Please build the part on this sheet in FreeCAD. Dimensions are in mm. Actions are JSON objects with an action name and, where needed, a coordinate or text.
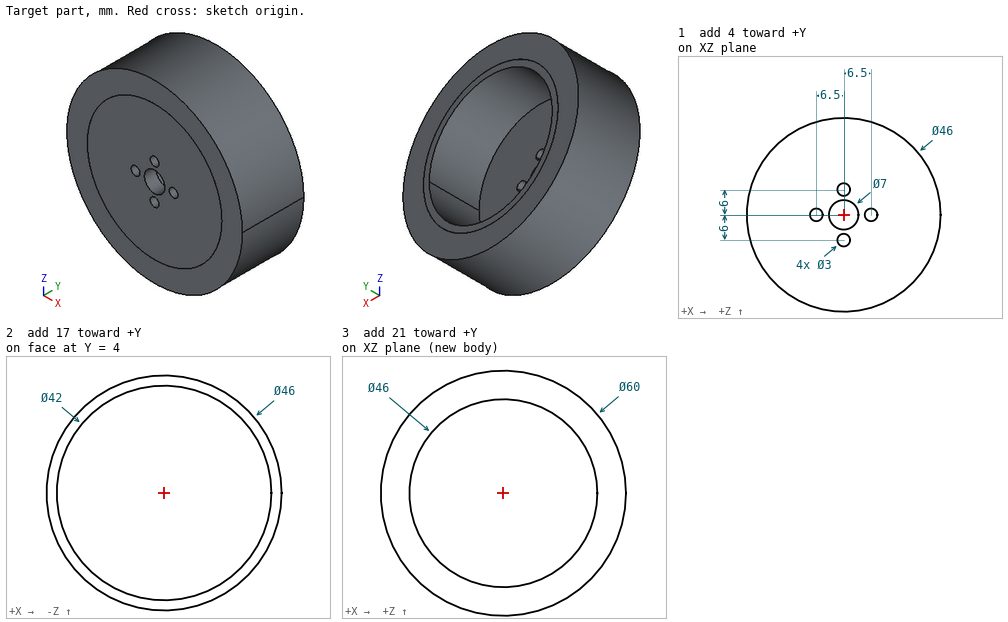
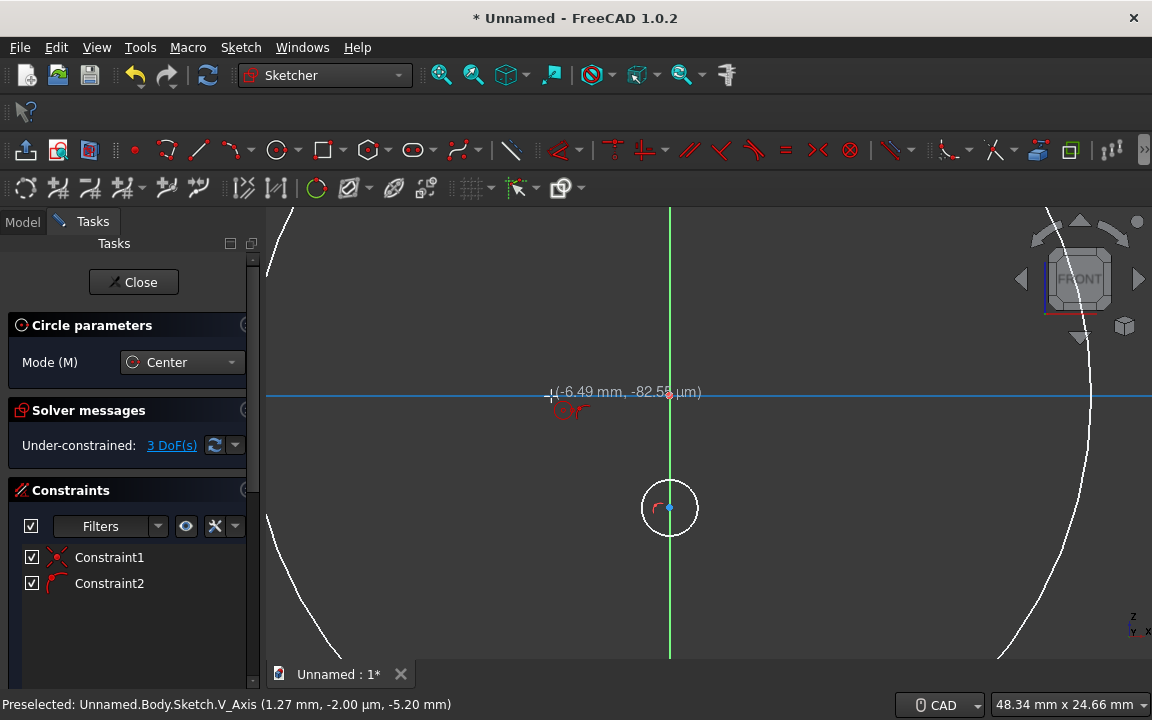
{"action": "scroll", "coordinate": [628, 449], "scroll_direction": "down", "scroll_amount": 6}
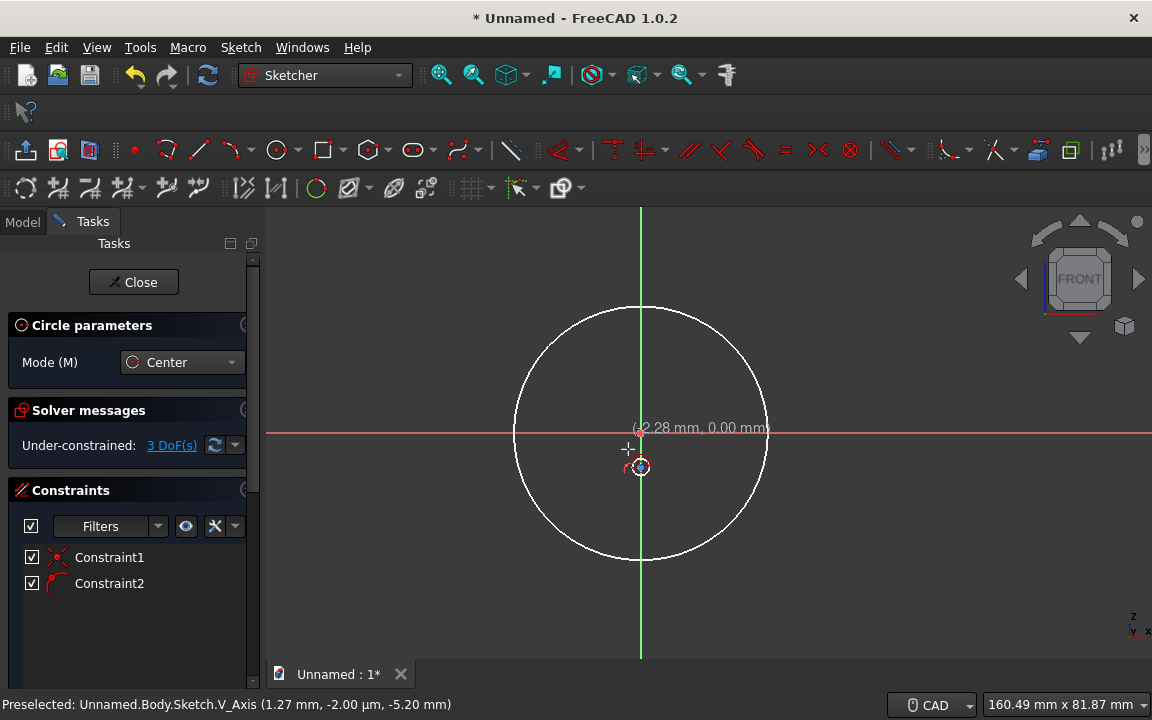
{"action": "left_click", "coordinate": [605, 433]}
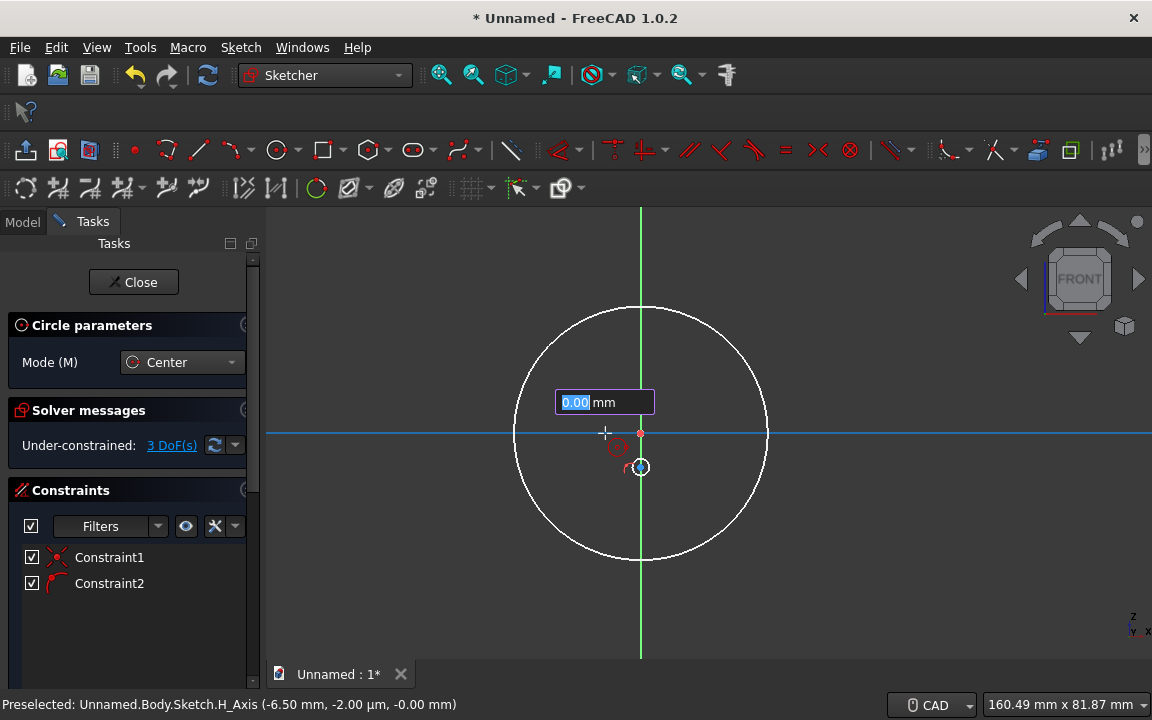
{"action": "scroll", "coordinate": [602, 441], "scroll_direction": "up", "scroll_amount": 4}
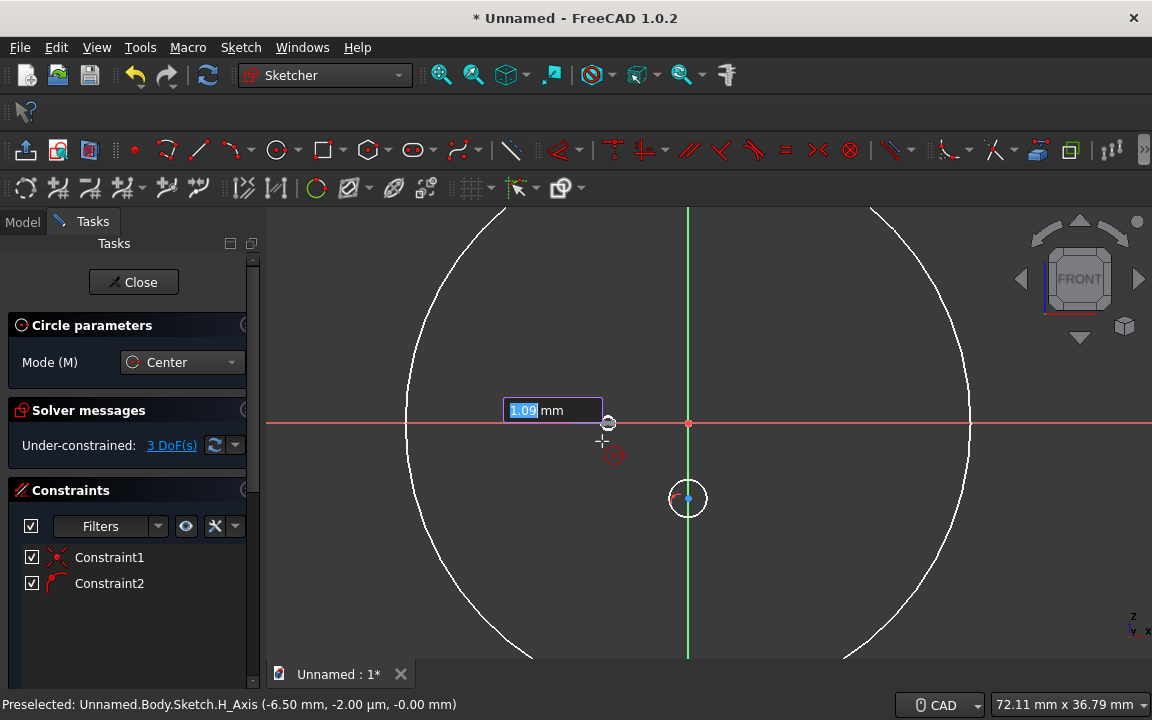
{"action": "left_click", "coordinate": [602, 441]}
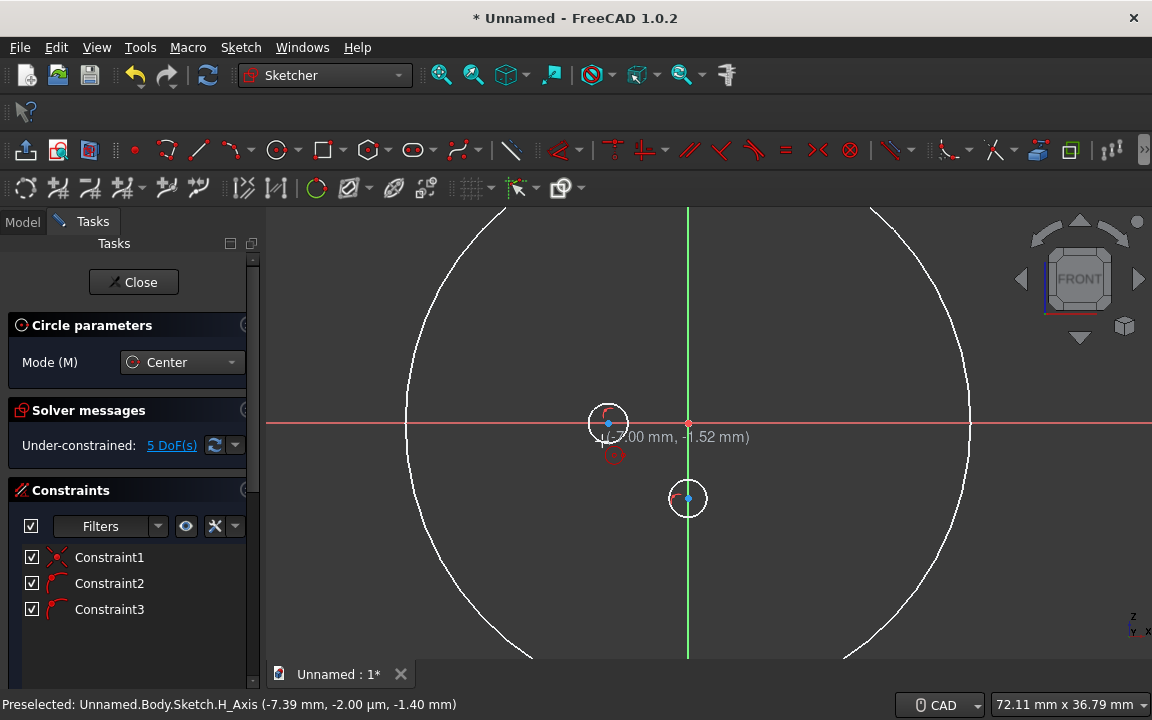
{"action": "scroll", "coordinate": [768, 423], "scroll_direction": "up", "scroll_amount": 2}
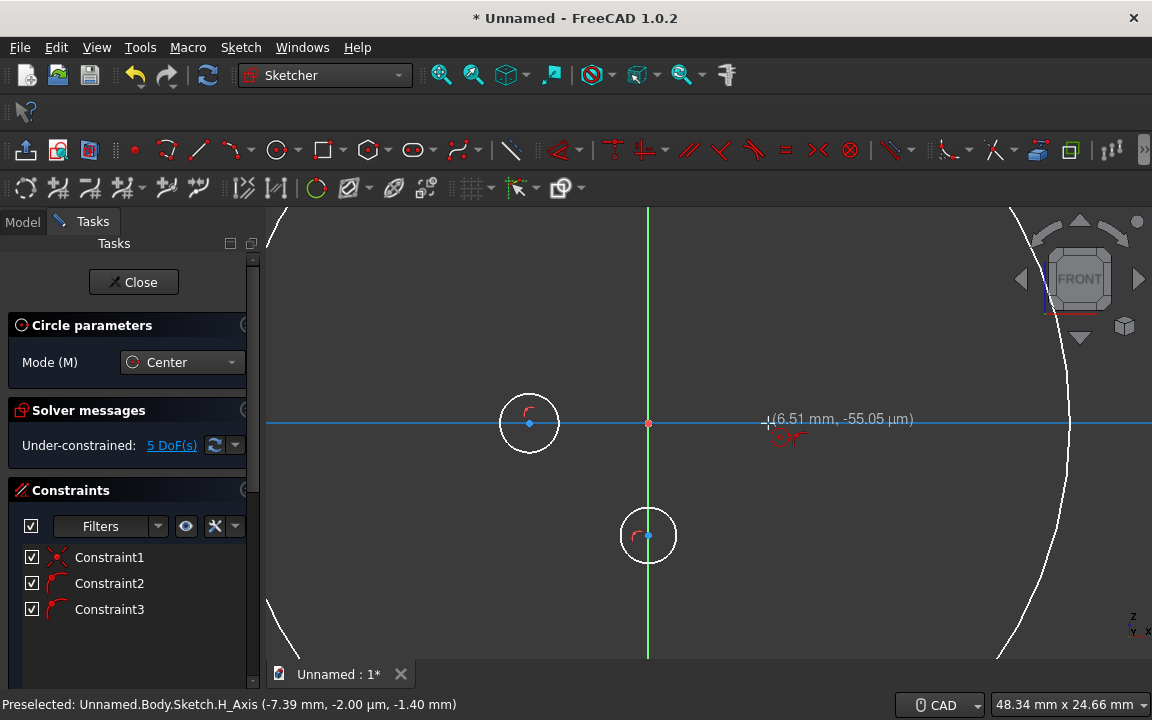
{"action": "scroll", "coordinate": [637, 437], "scroll_direction": "down", "scroll_amount": 6}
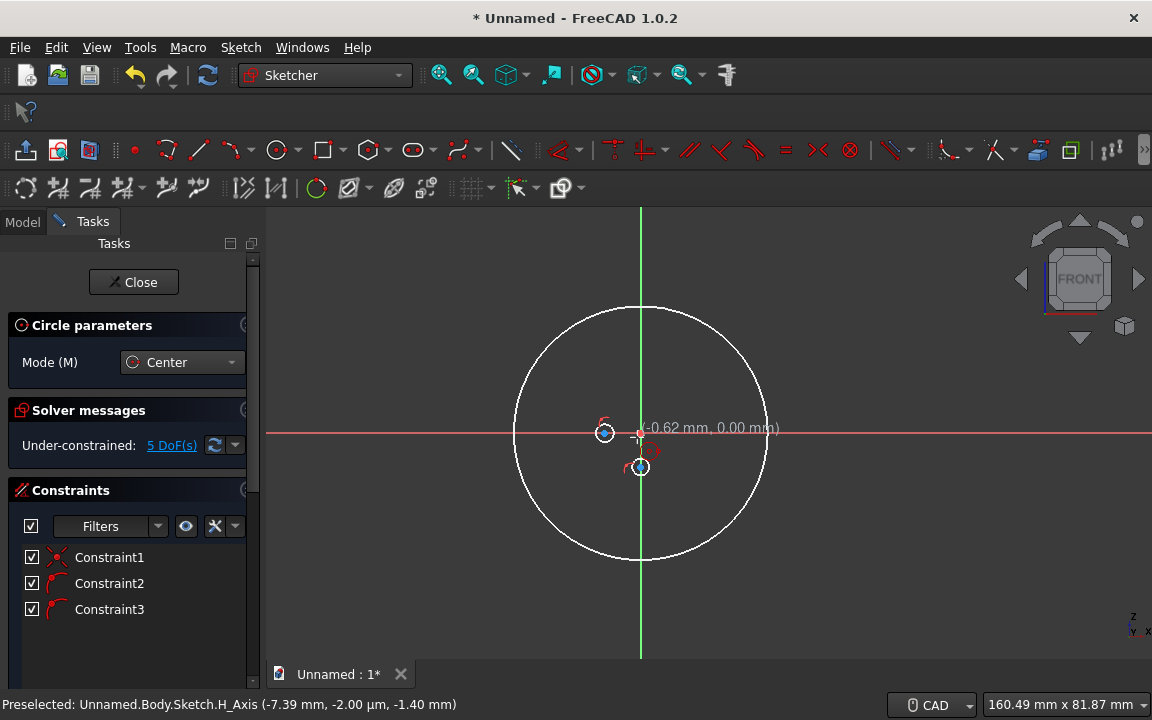
{"action": "left_click", "coordinate": [677, 433]}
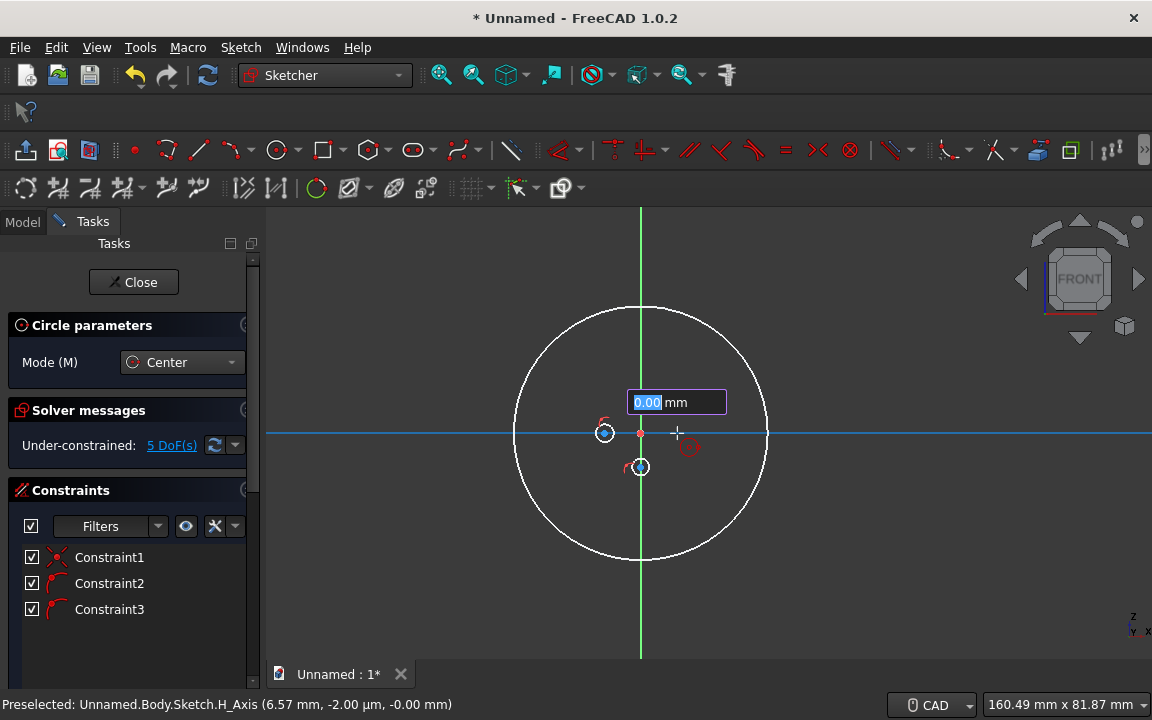
{"action": "scroll", "coordinate": [674, 441], "scroll_direction": "up", "scroll_amount": 4}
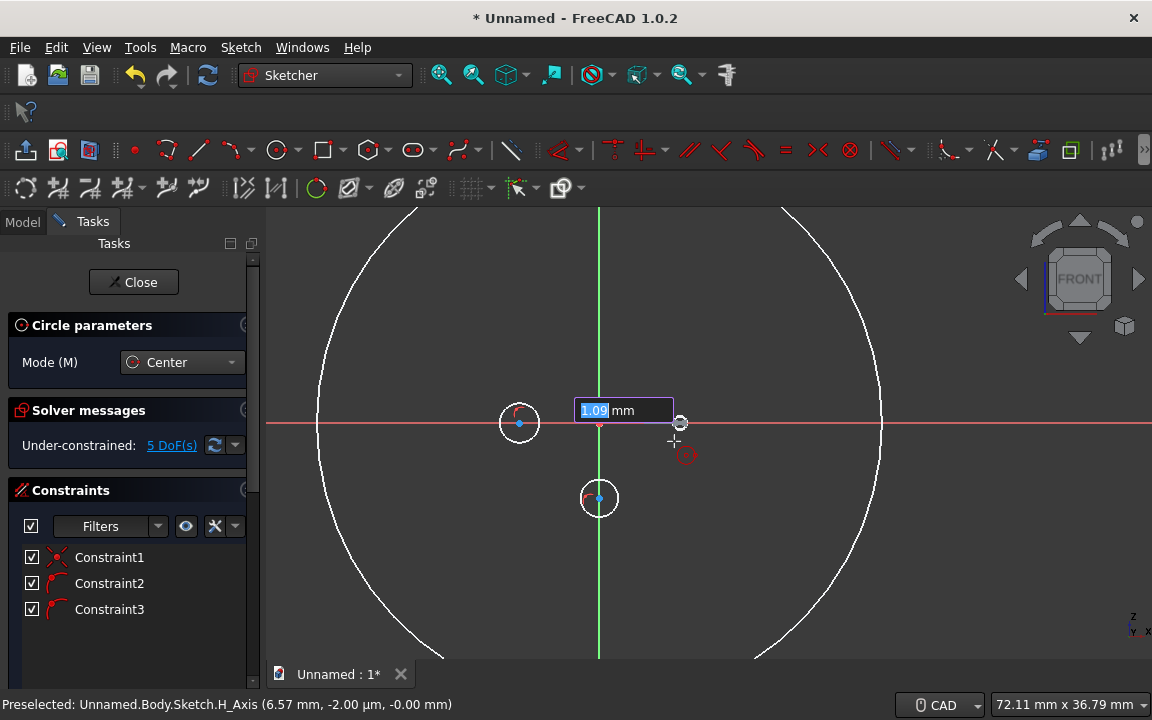
{"action": "left_click", "coordinate": [673, 440]}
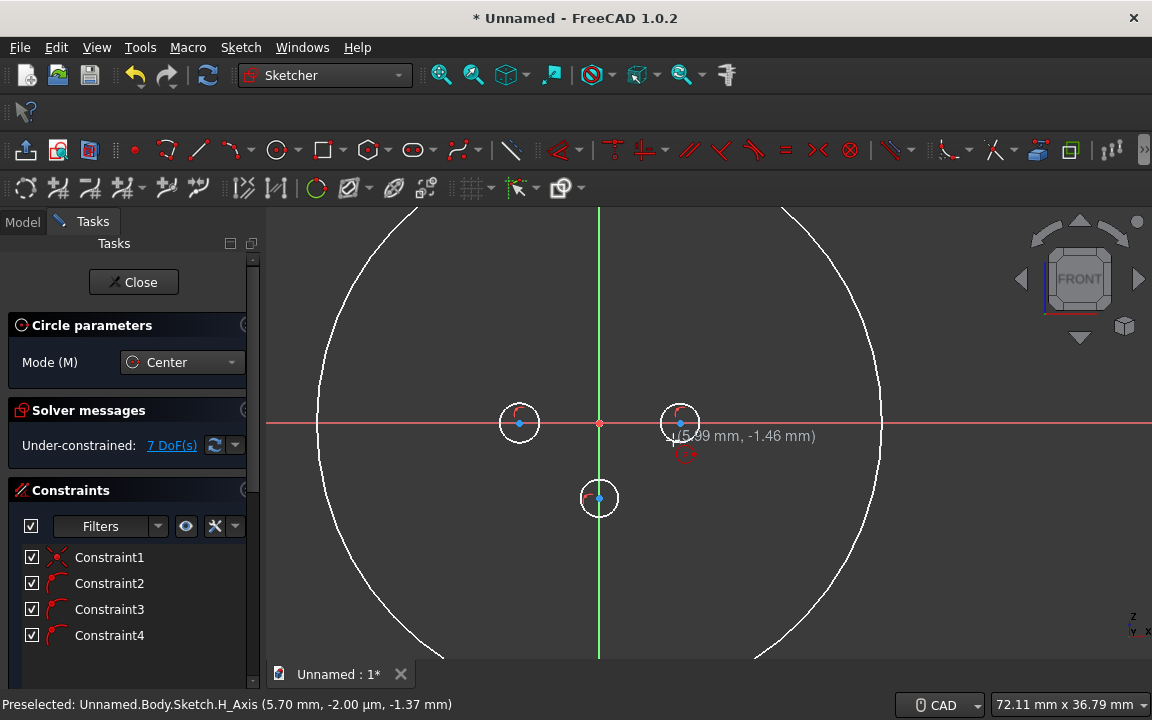
{"action": "left_click", "coordinate": [599, 423]}
{"action": "left_click", "coordinate": [630, 393]}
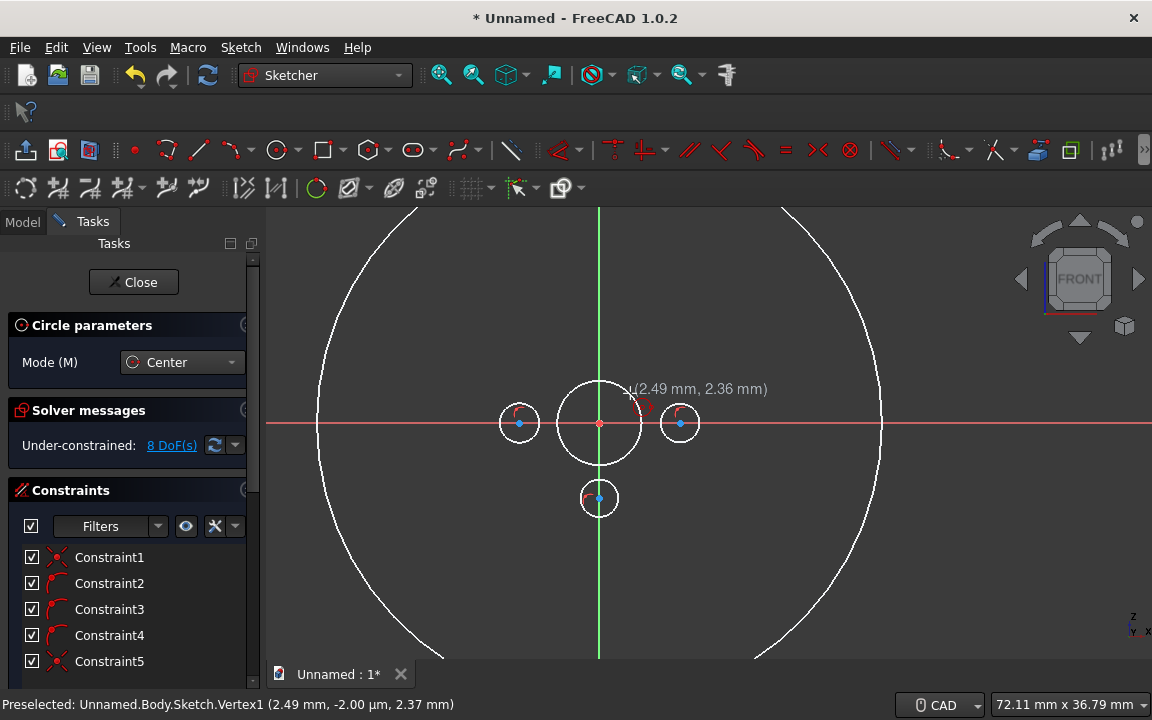
{"action": "scroll", "coordinate": [599, 349], "scroll_direction": "up", "scroll_amount": 2}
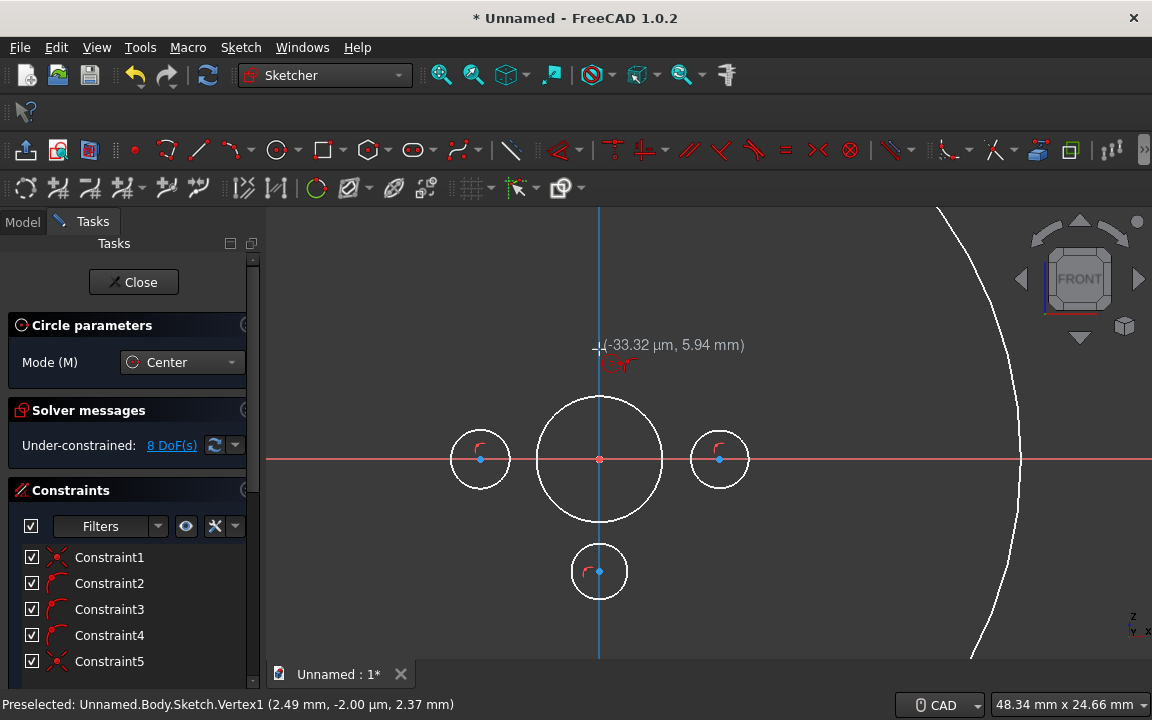
{"action": "scroll", "coordinate": [658, 422], "scroll_direction": "down", "scroll_amount": 6}